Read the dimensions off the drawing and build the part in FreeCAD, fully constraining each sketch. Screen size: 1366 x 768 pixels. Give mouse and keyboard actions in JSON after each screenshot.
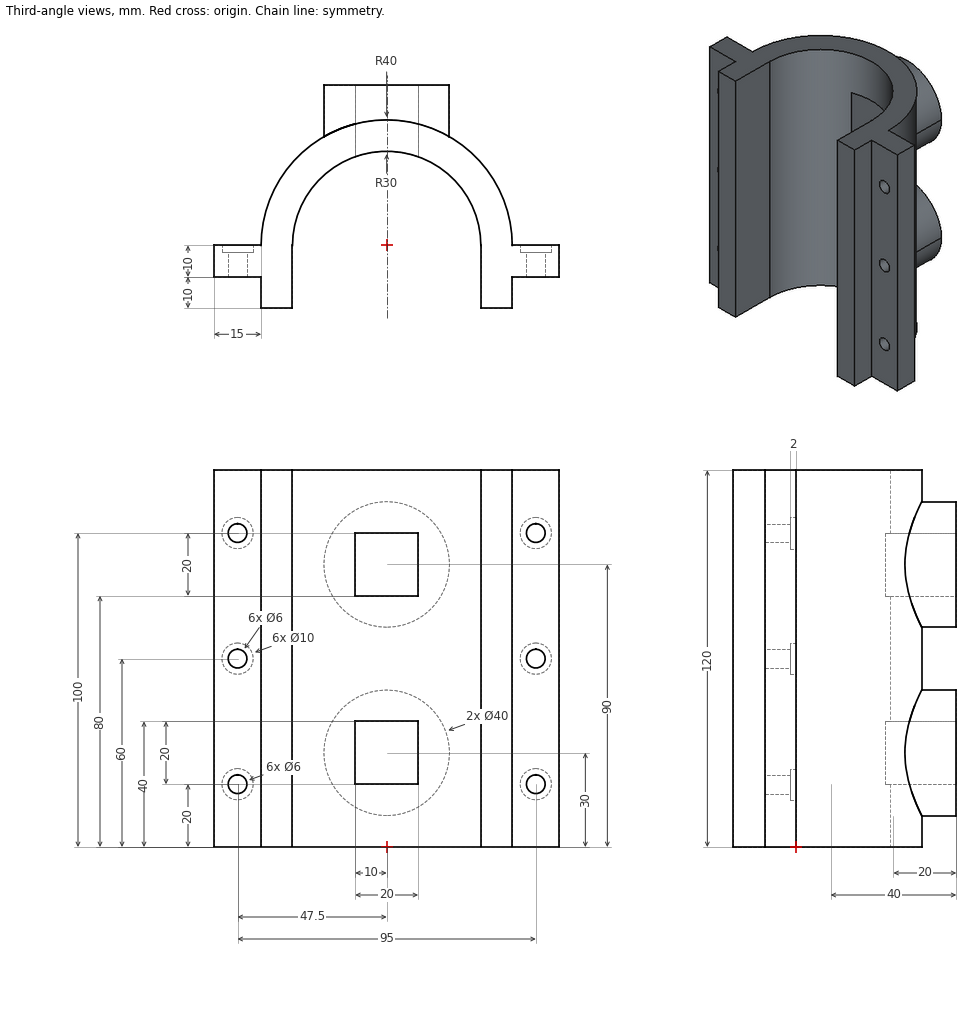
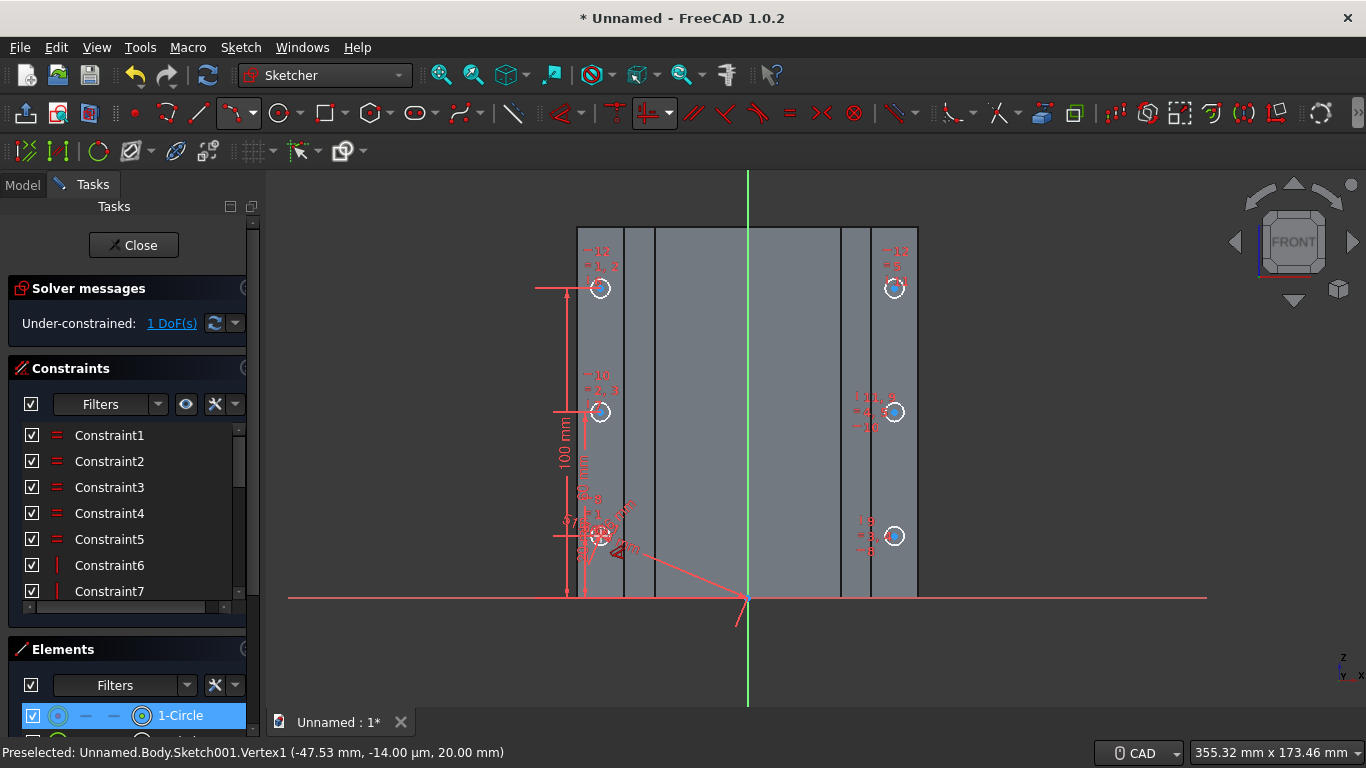
{"action": "left_click", "coordinate": [895, 536]}
{"action": "left_click", "coordinate": [680, 570]}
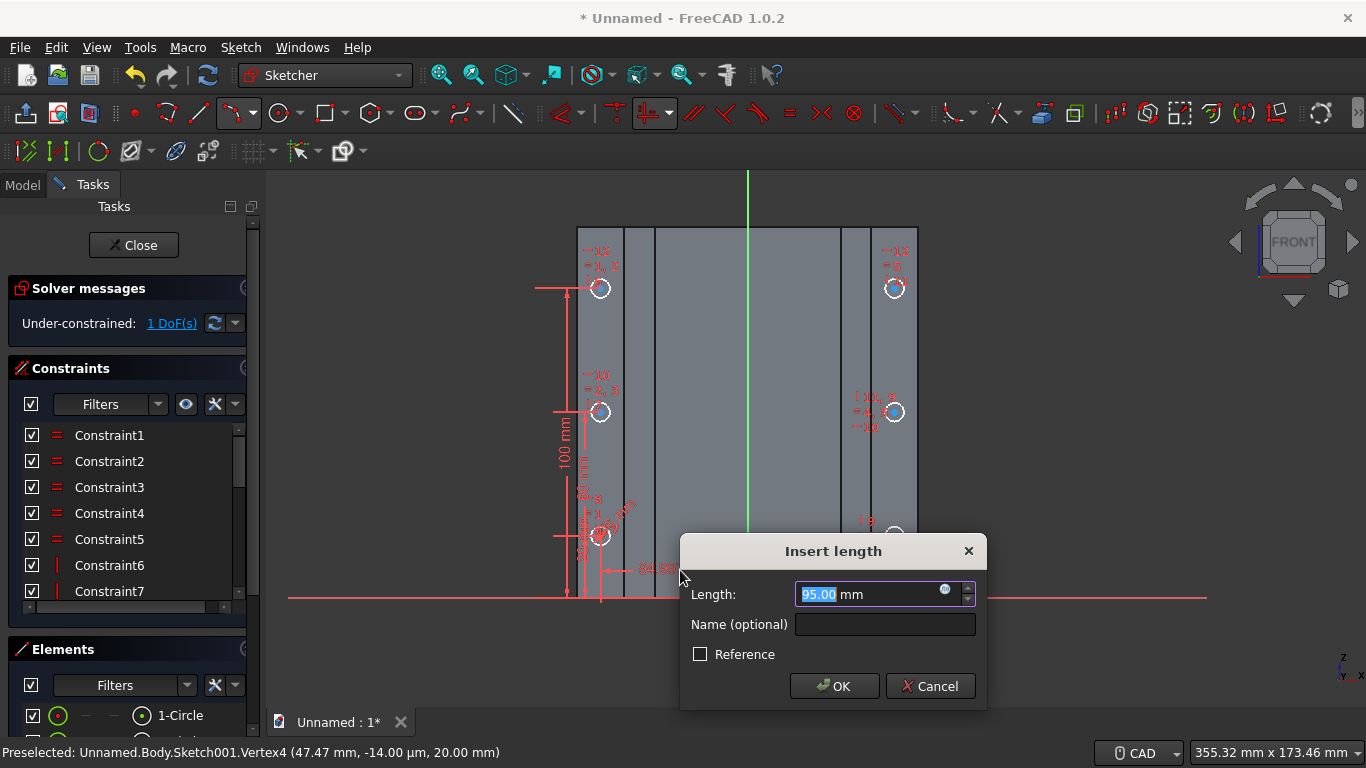
{"action": "type", "text": "95"}
{"action": "key", "text": "Return"}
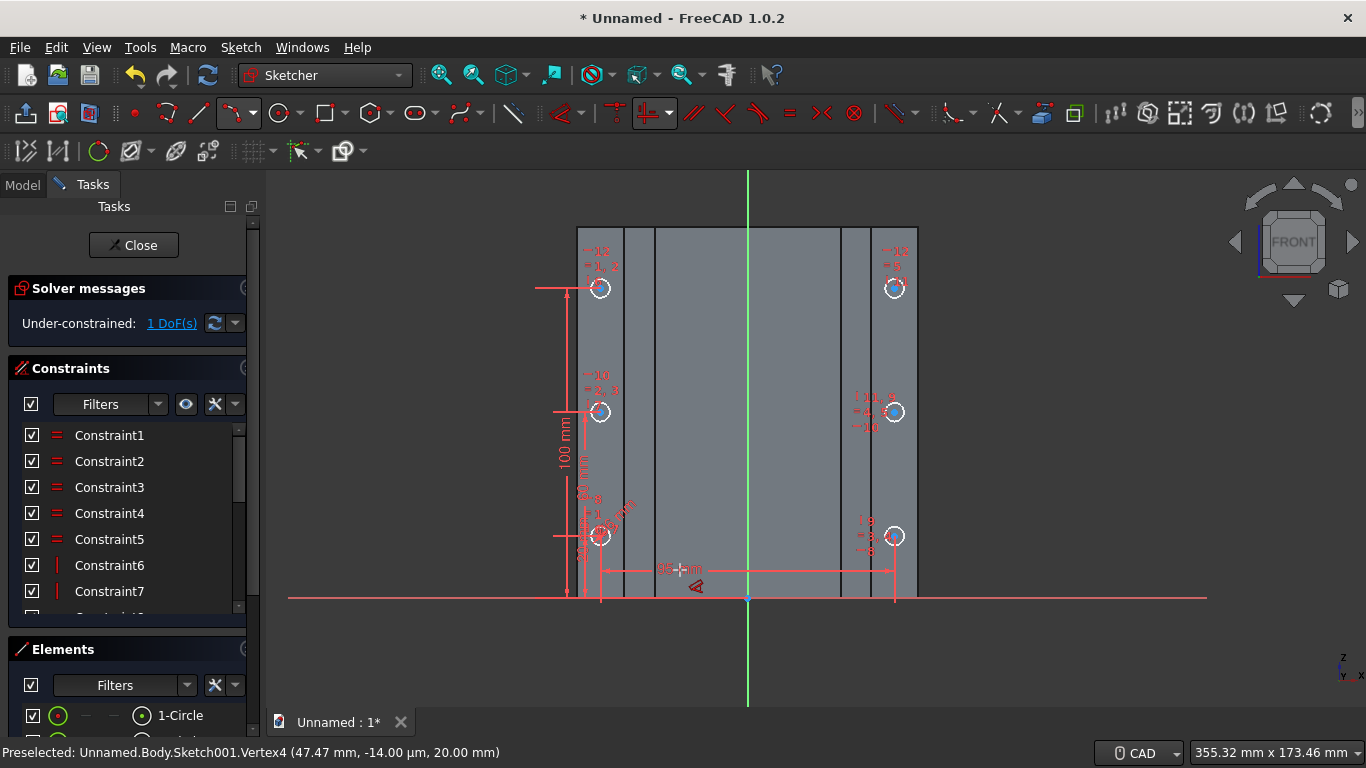
{"action": "left_click", "coordinate": [601, 536]}
{"action": "left_click", "coordinate": [674, 632]}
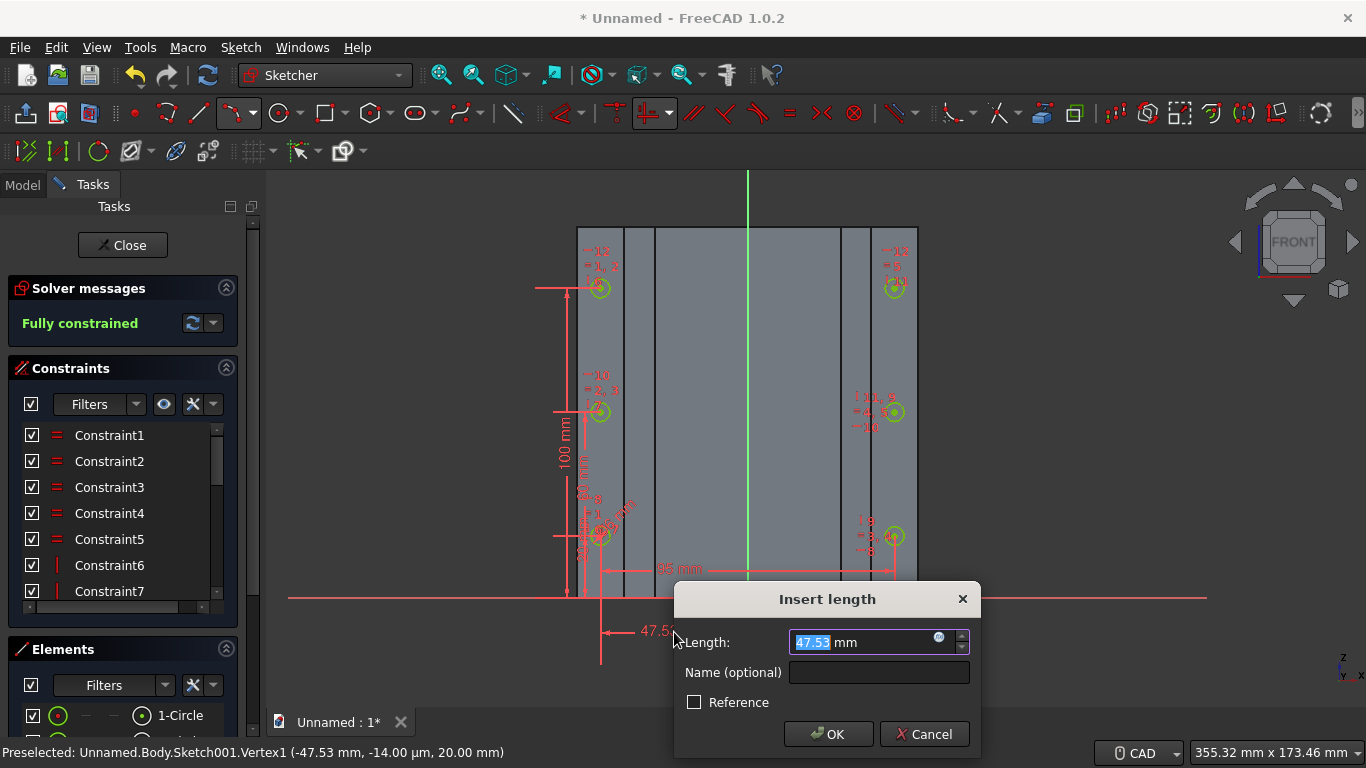
{"action": "type", "text": "47.5"}
{"action": "key", "text": "Return"}
{"action": "key", "text": "Escape"}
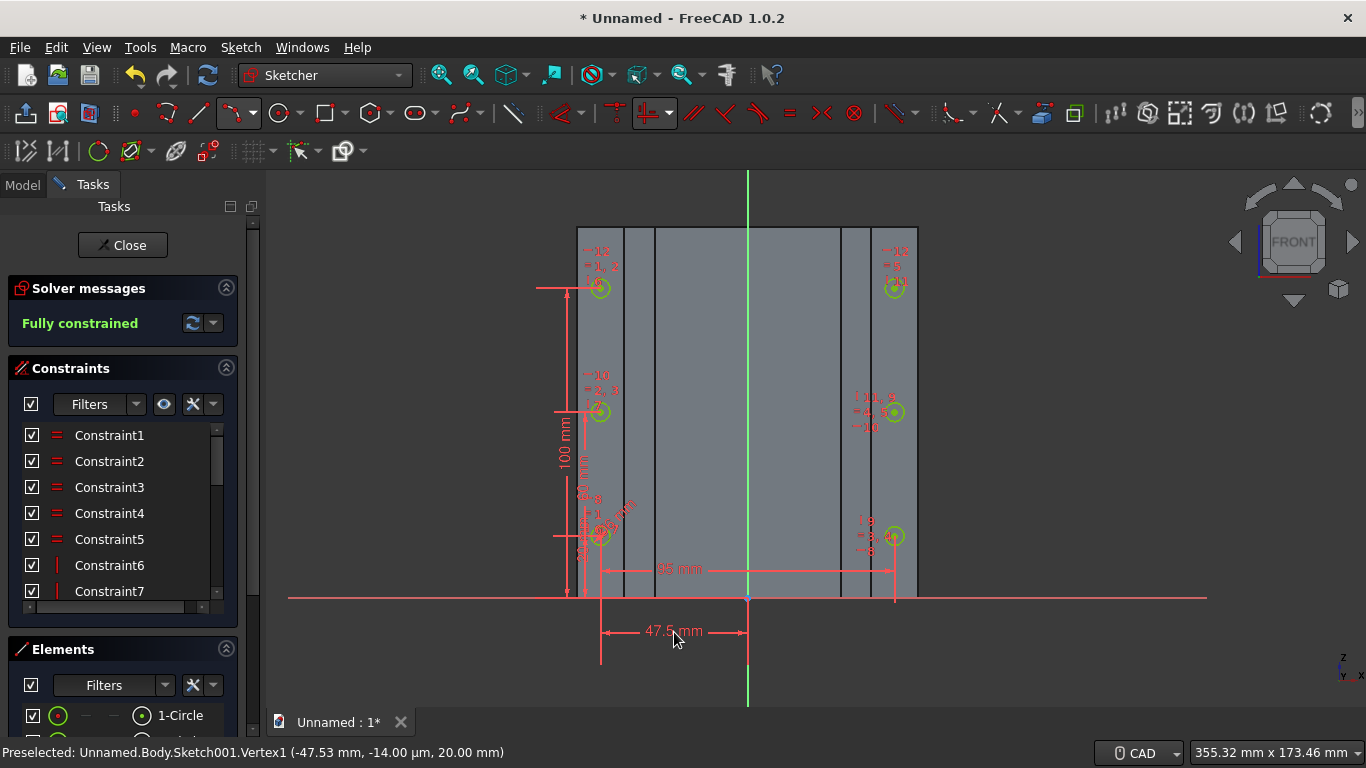
{"action": "left_click", "coordinate": [123, 245]}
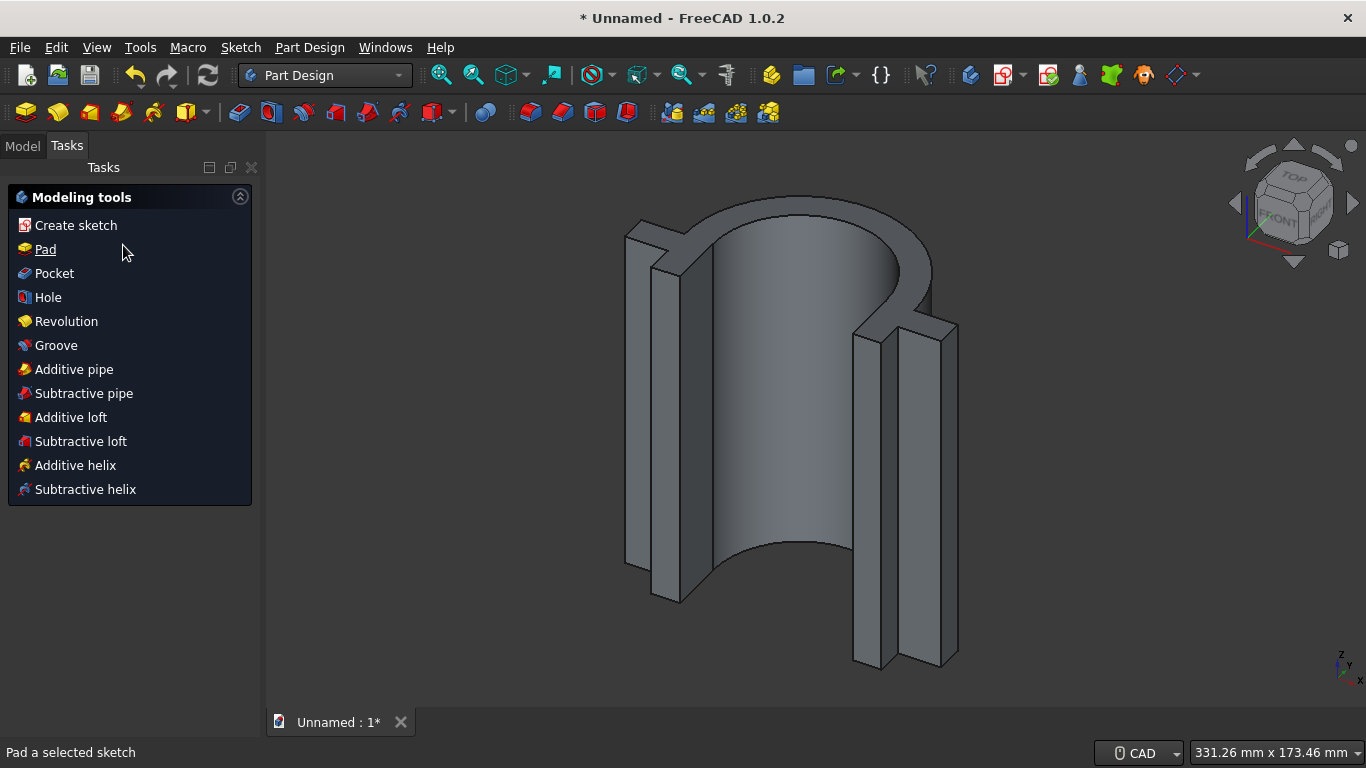
{"action": "left_click", "coordinate": [240, 112]}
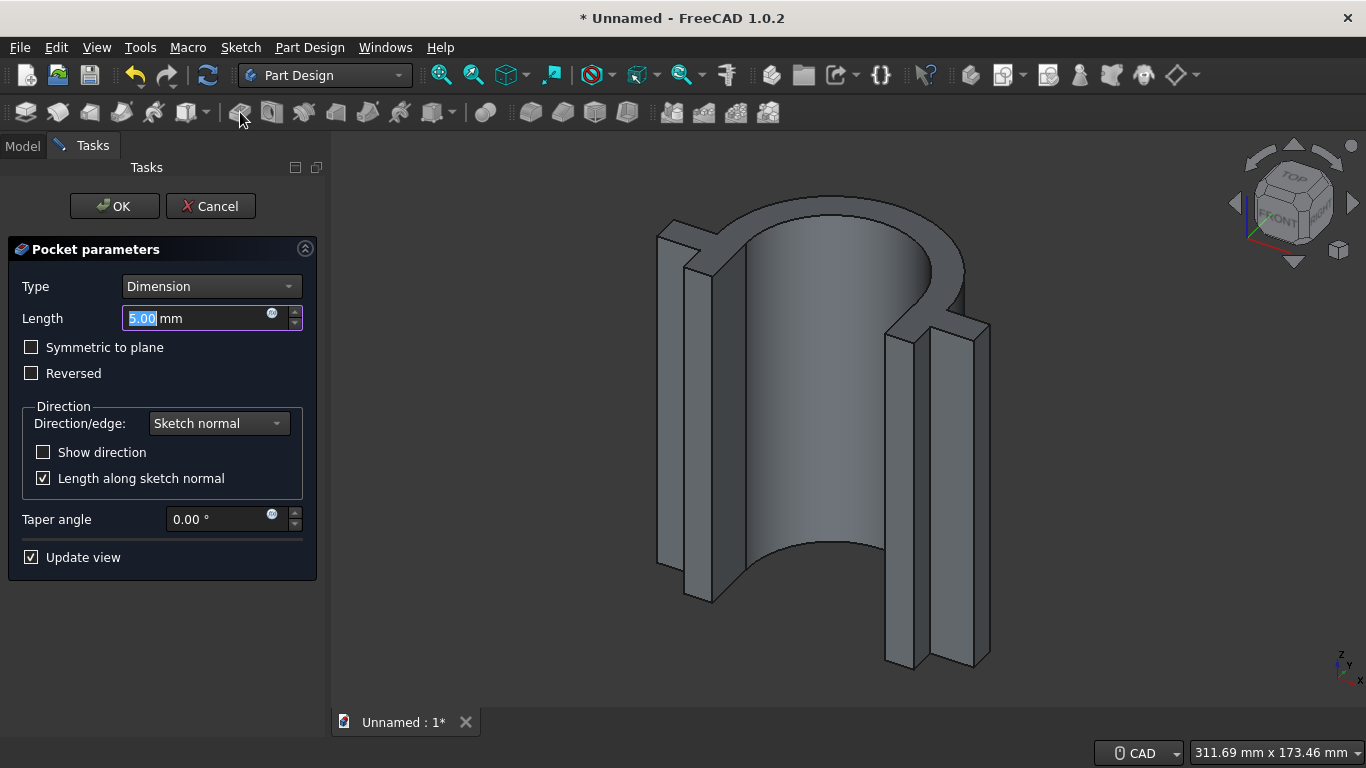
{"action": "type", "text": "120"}
{"action": "key", "text": "Tab"}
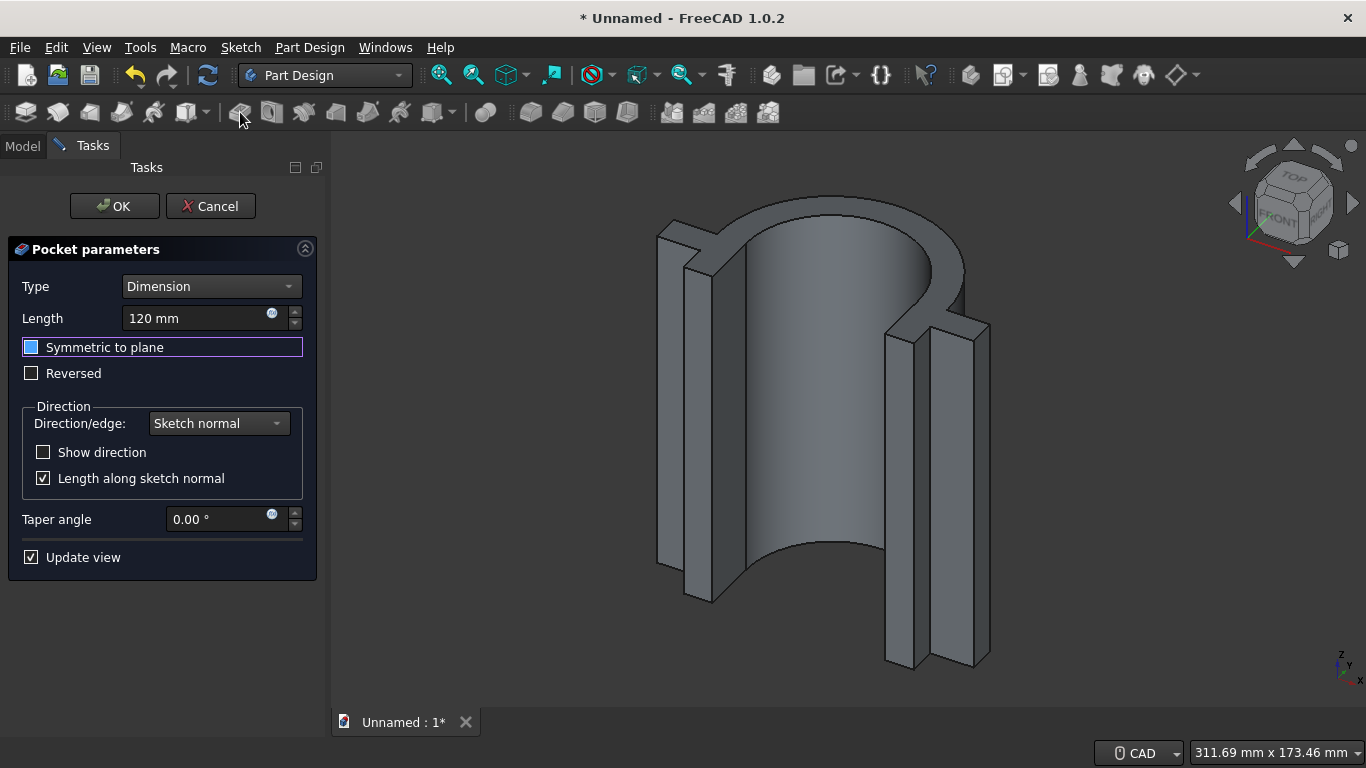
{"action": "left_click", "coordinate": [30, 373]}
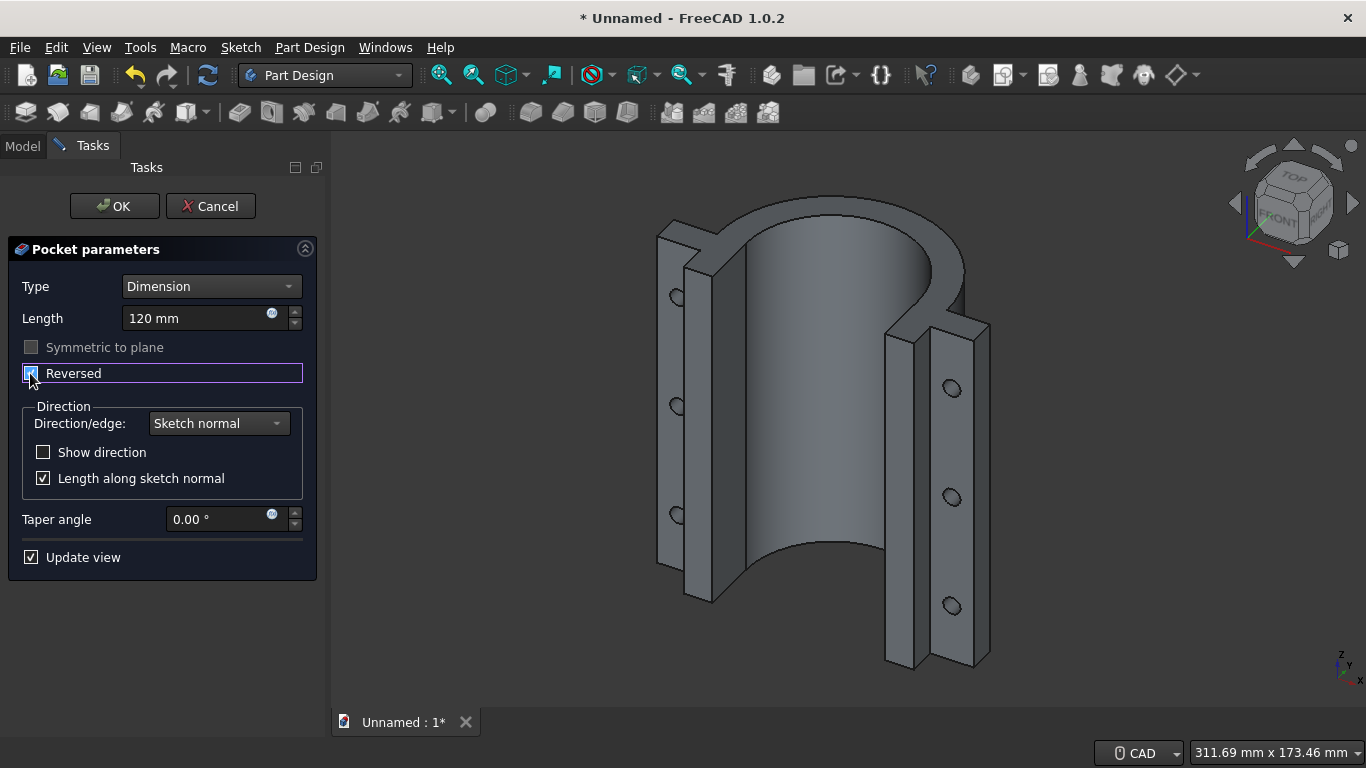
{"action": "left_click", "coordinate": [115, 206]}